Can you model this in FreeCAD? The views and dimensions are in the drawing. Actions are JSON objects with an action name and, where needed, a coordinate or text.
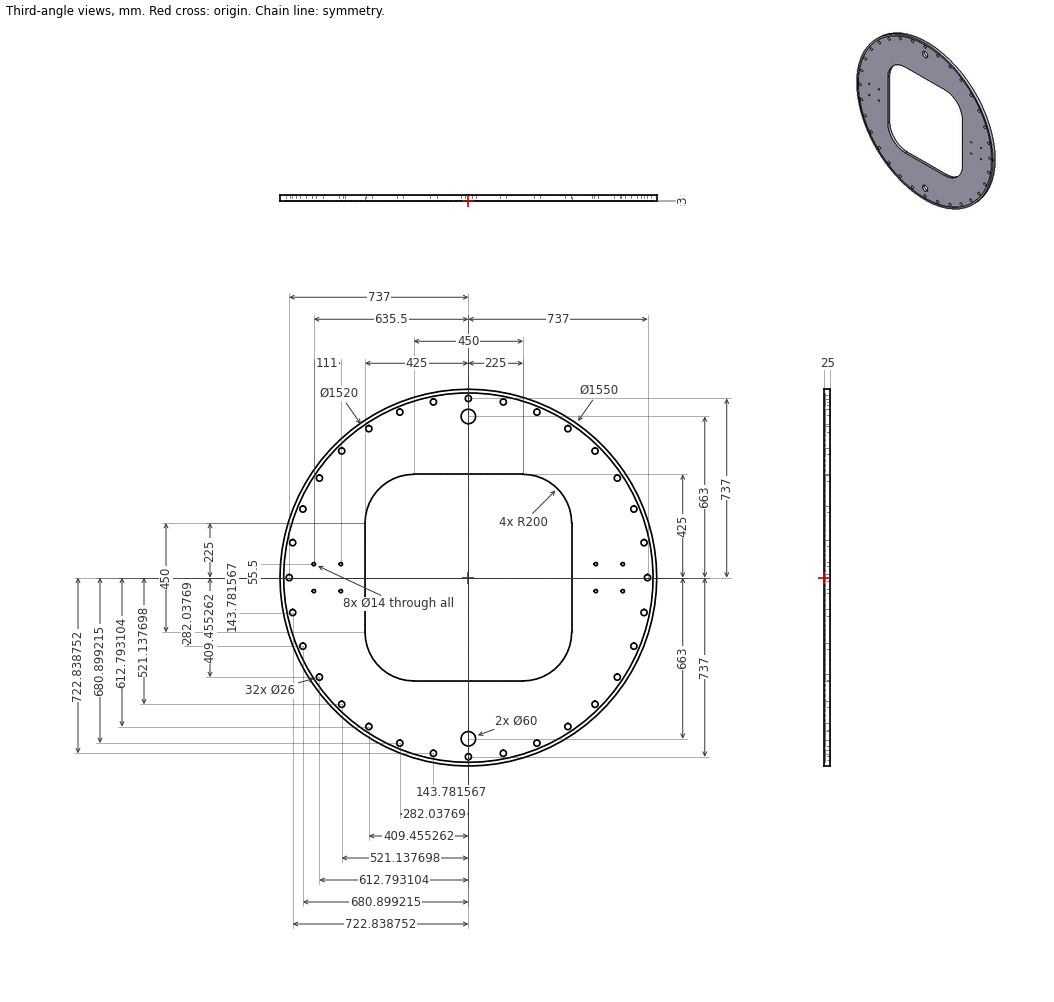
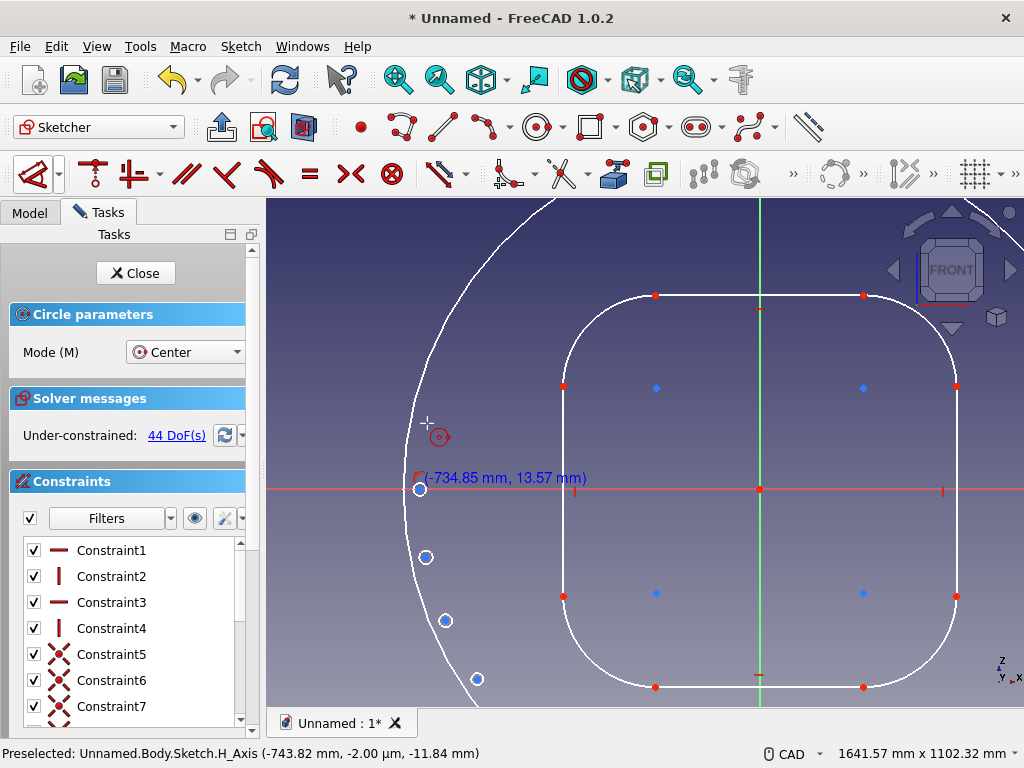
{"action": "left_click", "coordinate": [426, 423]}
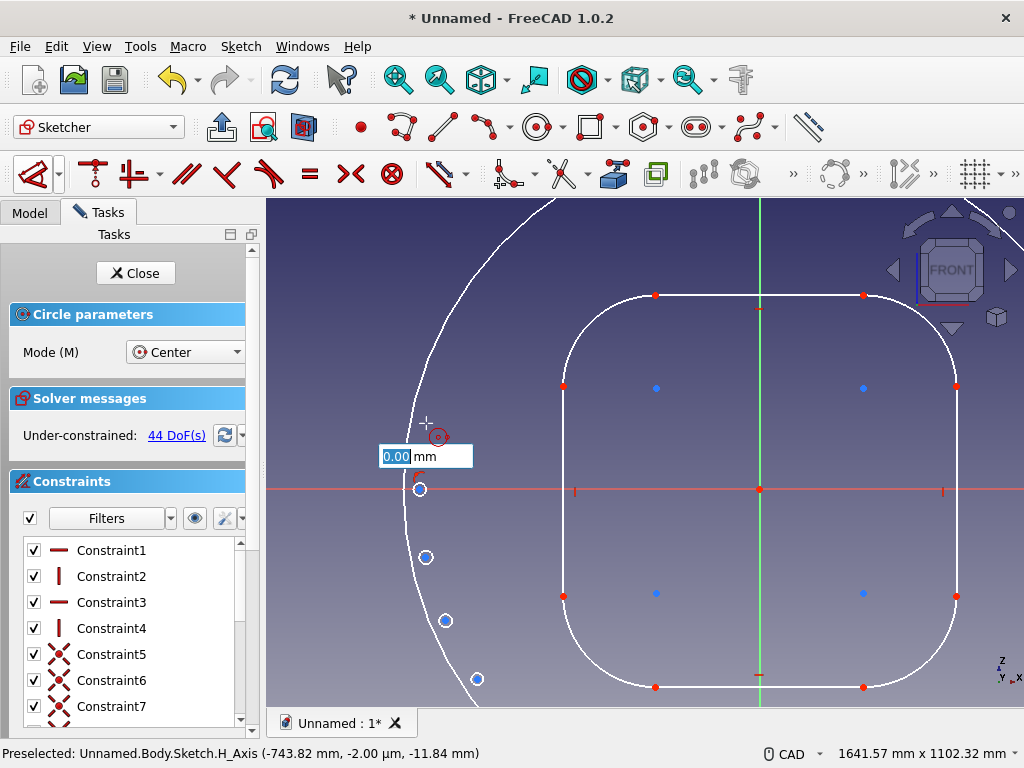
{"action": "scroll", "coordinate": [430, 419], "scroll_direction": "up", "scroll_amount": 5}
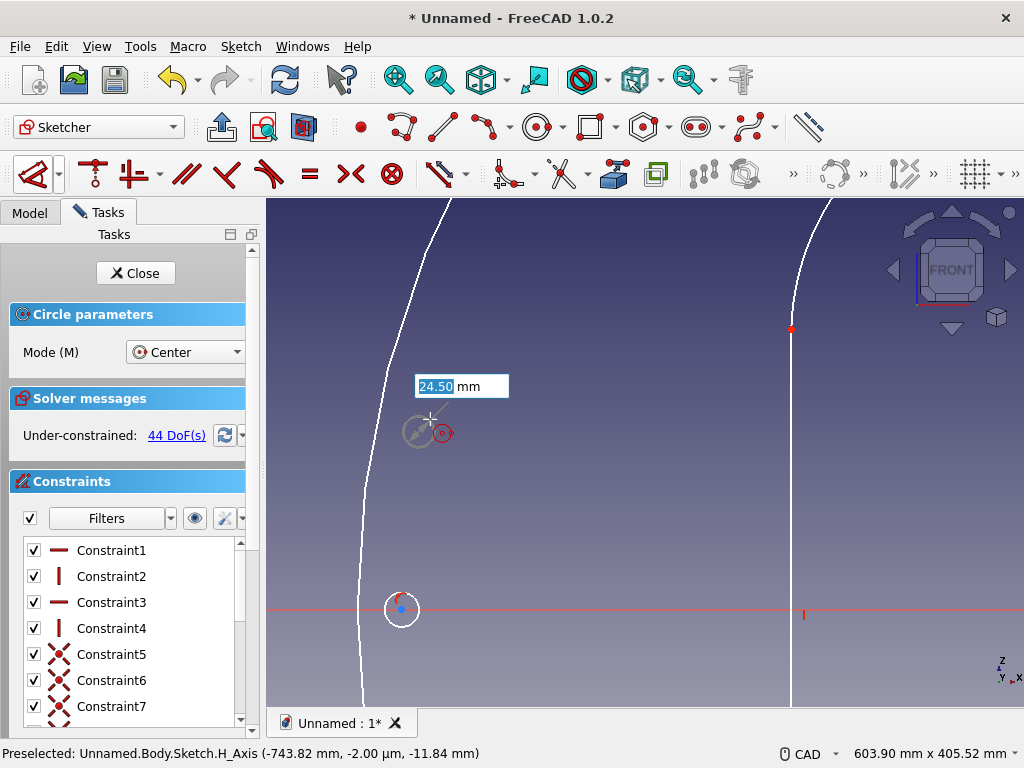
{"action": "left_click", "coordinate": [430, 418]}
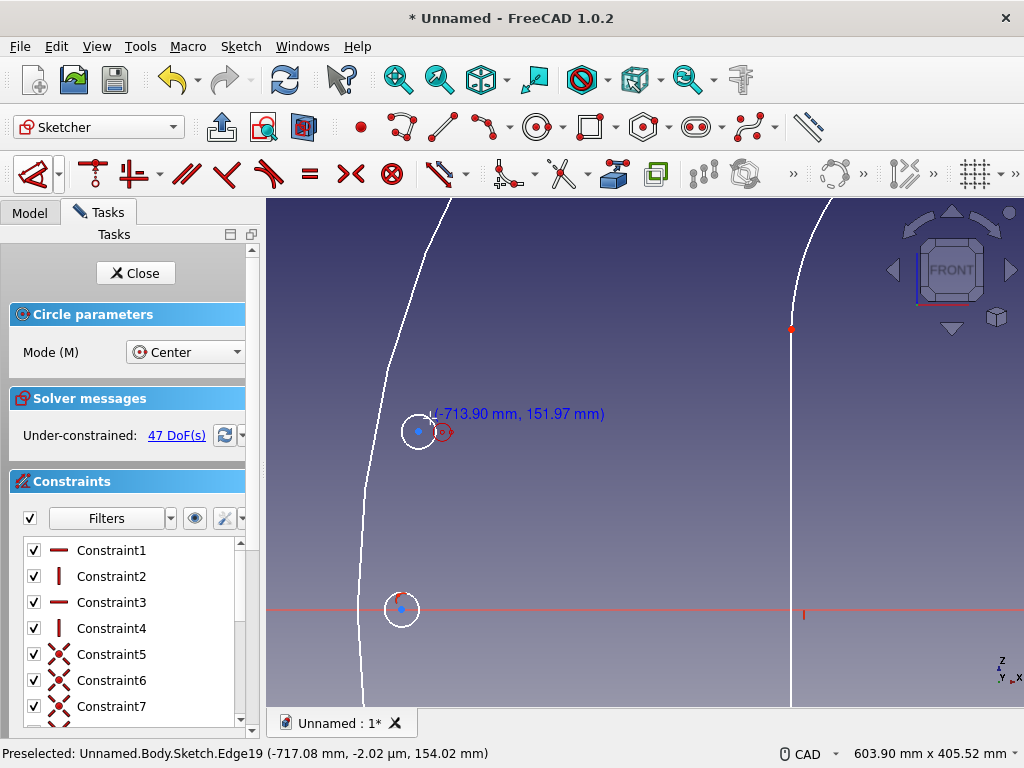
{"action": "scroll", "coordinate": [471, 256], "scroll_direction": "up", "scroll_amount": 2}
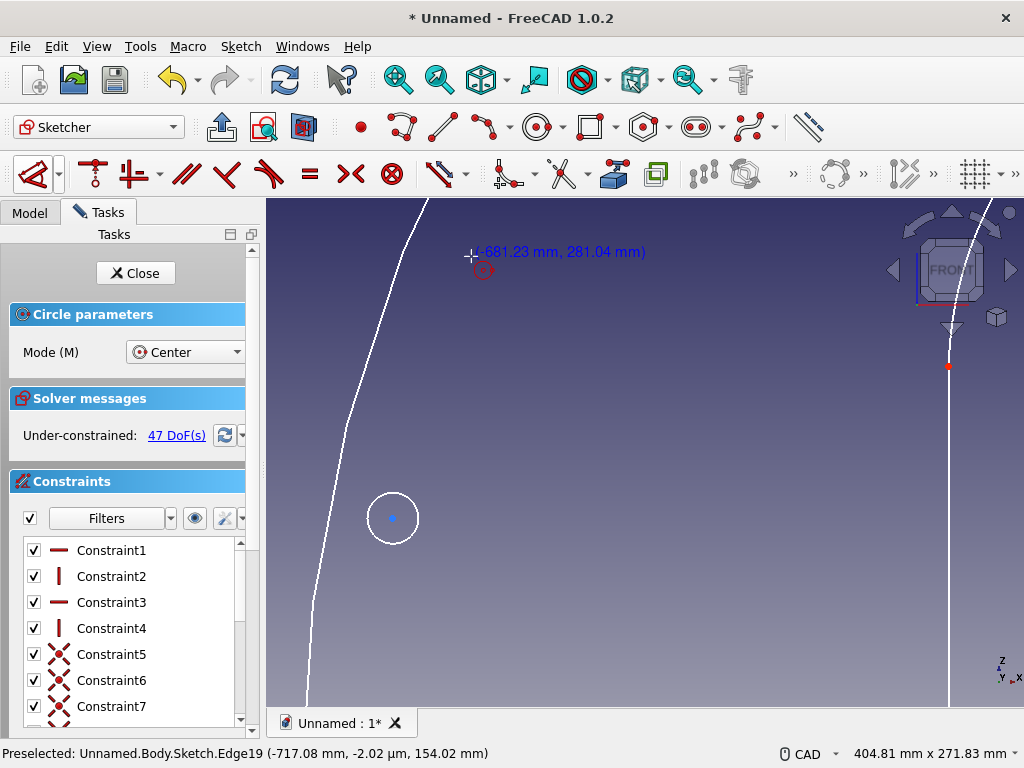
{"action": "scroll", "coordinate": [431, 411], "scroll_direction": "down", "scroll_amount": 11}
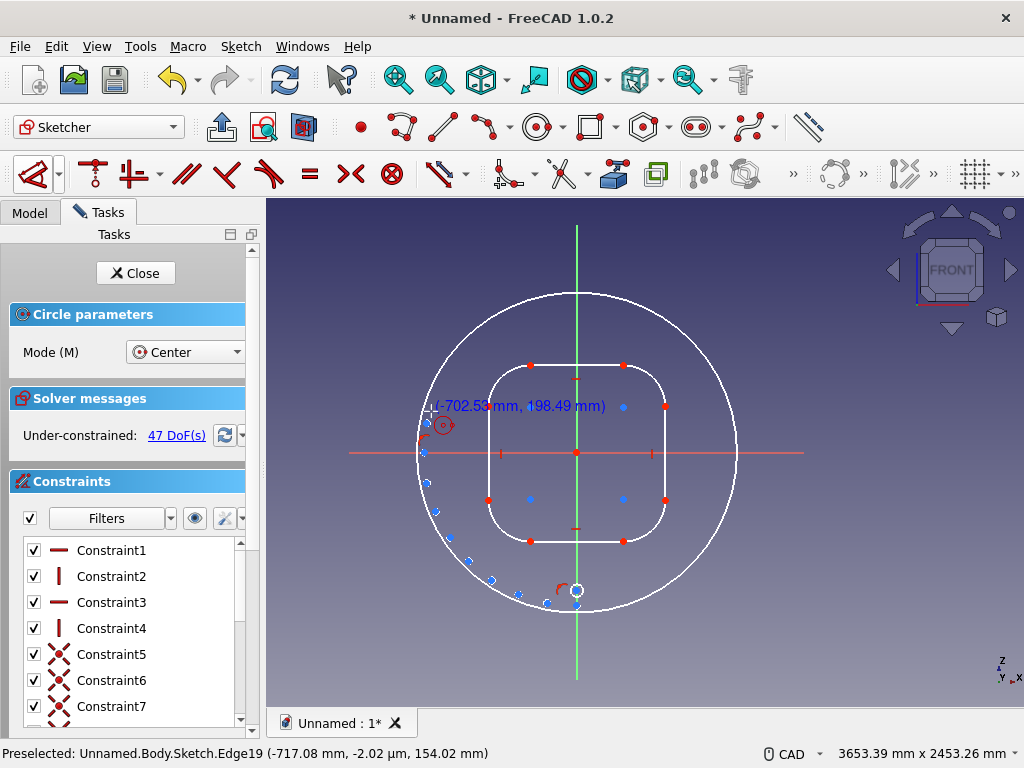
{"action": "scroll", "coordinate": [436, 394], "scroll_direction": "up", "scroll_amount": 4}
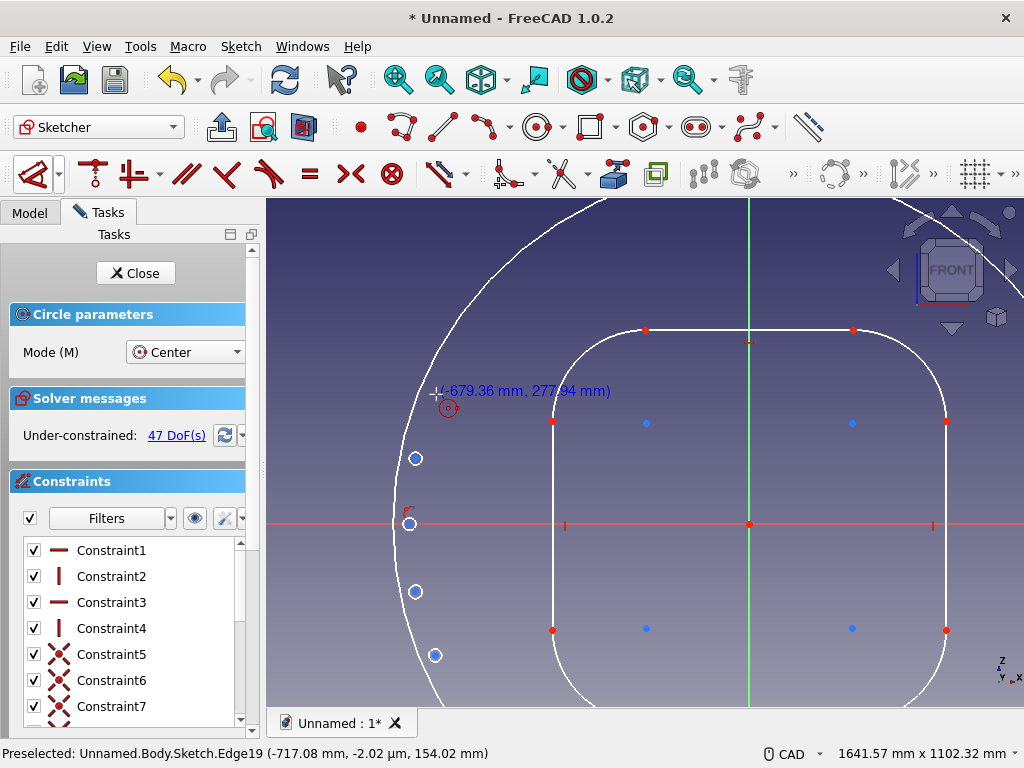
{"action": "left_click", "coordinate": [435, 394]}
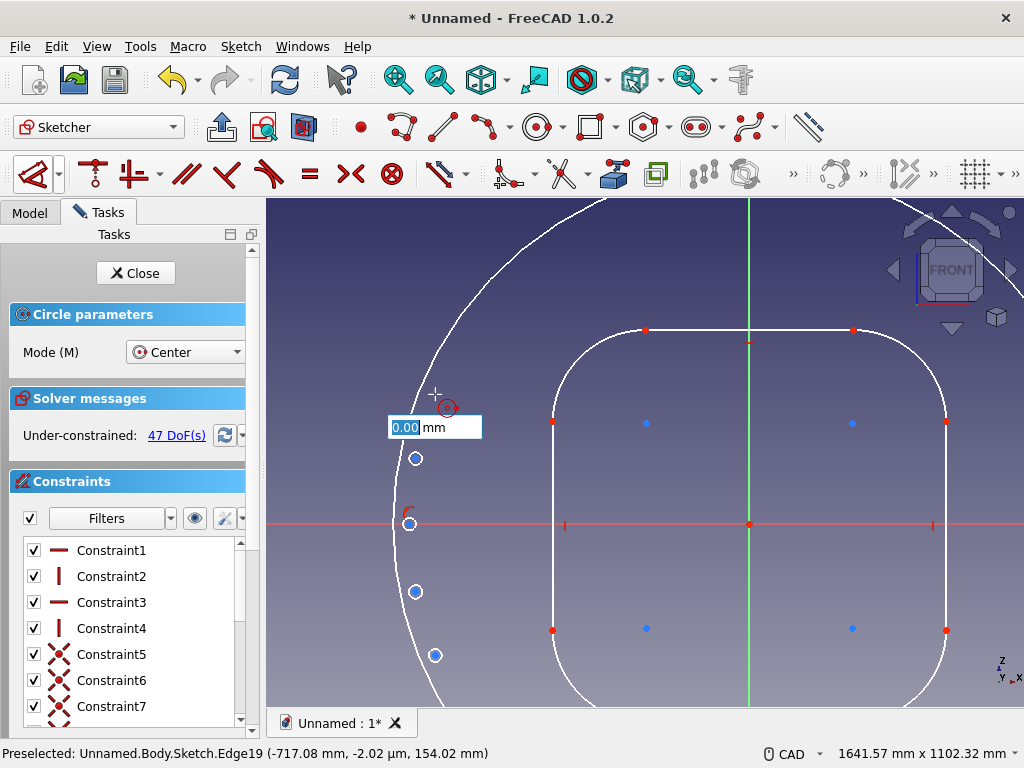
{"action": "scroll", "coordinate": [439, 390], "scroll_direction": "up", "scroll_amount": 5}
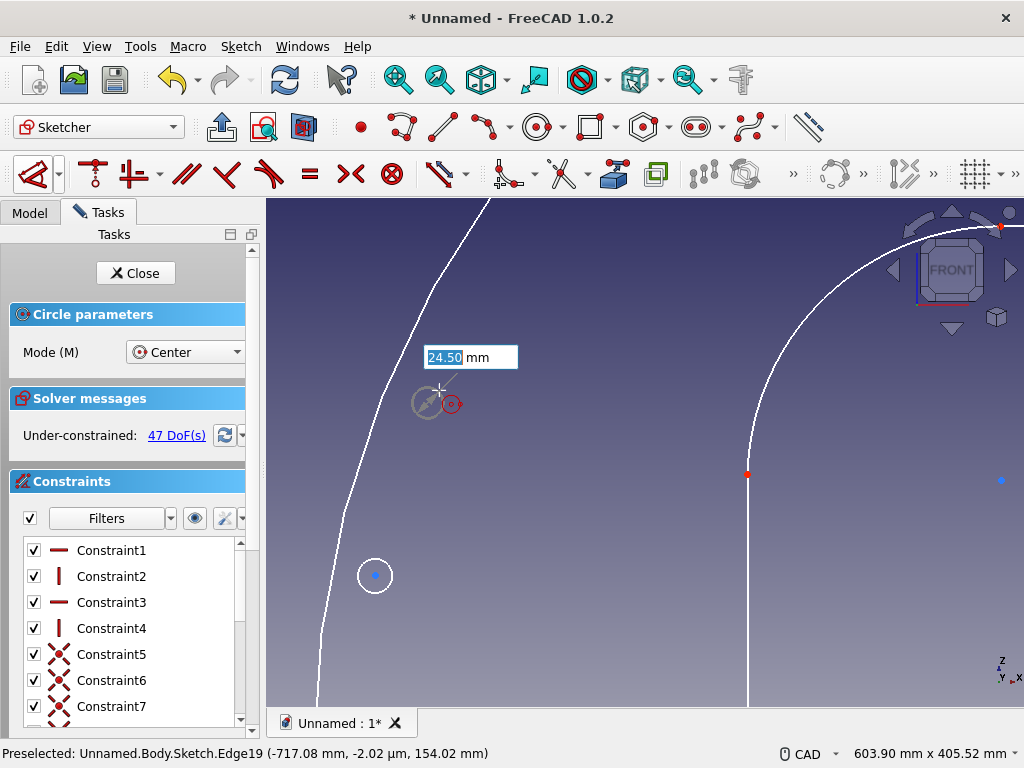
{"action": "left_click", "coordinate": [439, 388]}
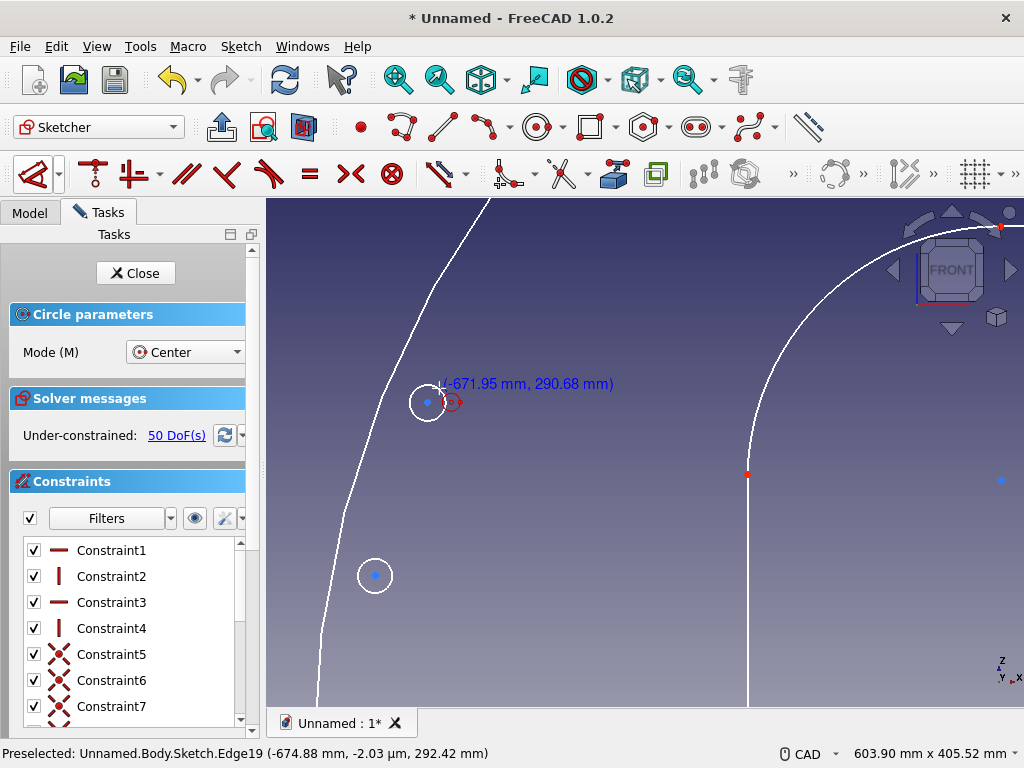
{"action": "scroll", "coordinate": [513, 240], "scroll_direction": "up", "scroll_amount": 2}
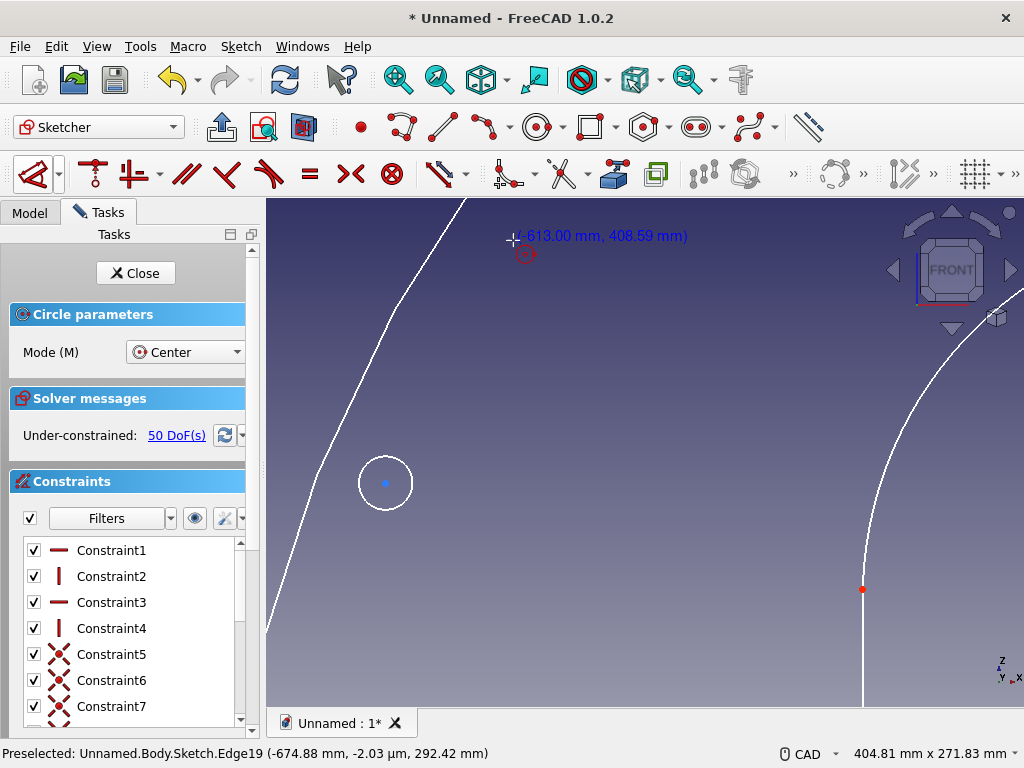
{"action": "scroll", "coordinate": [441, 383], "scroll_direction": "down", "scroll_amount": 11}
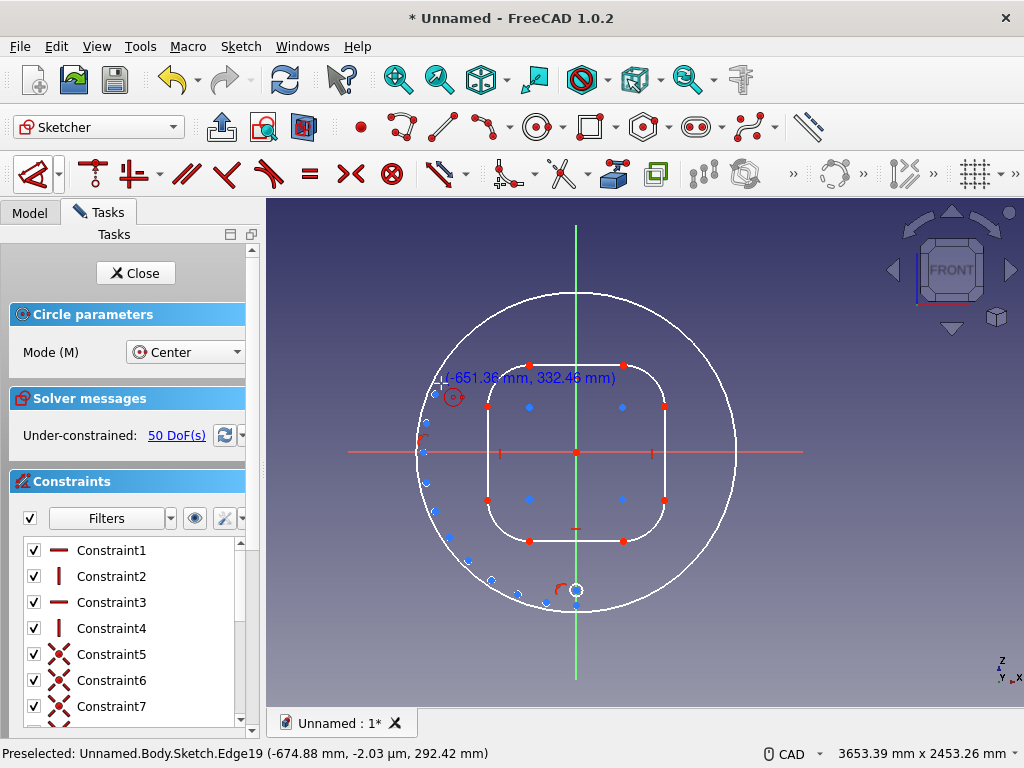
{"action": "scroll", "coordinate": [449, 367], "scroll_direction": "up", "scroll_amount": 4}